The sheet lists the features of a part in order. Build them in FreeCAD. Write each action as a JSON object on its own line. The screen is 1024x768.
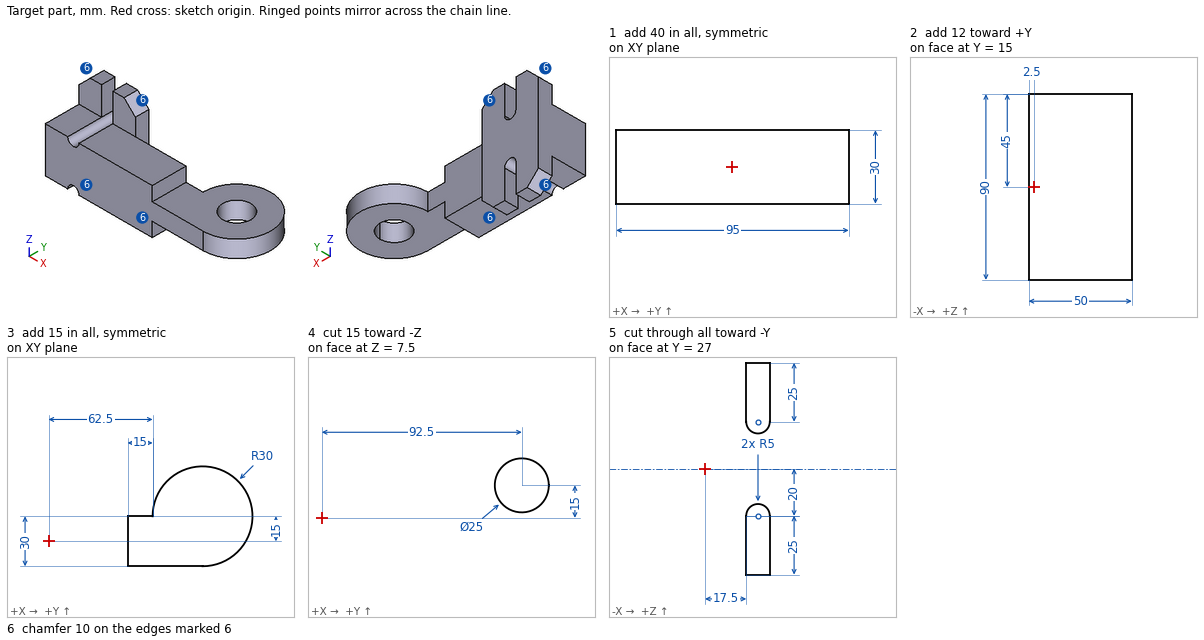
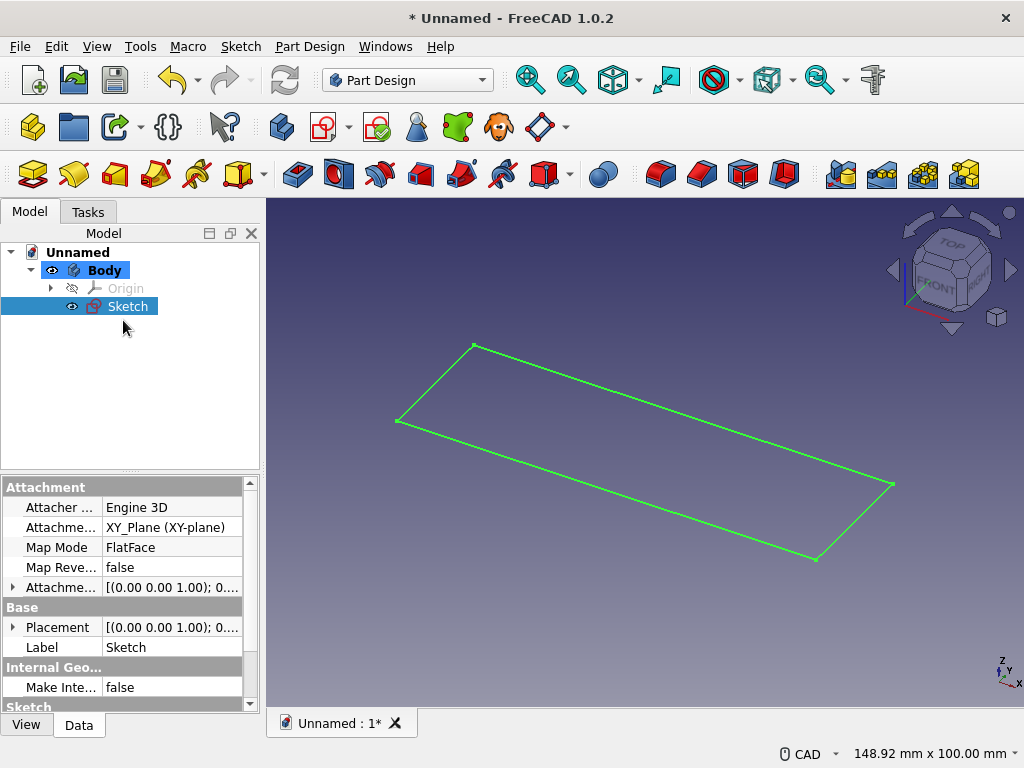
{"action": "left_click", "coordinate": [33, 174]}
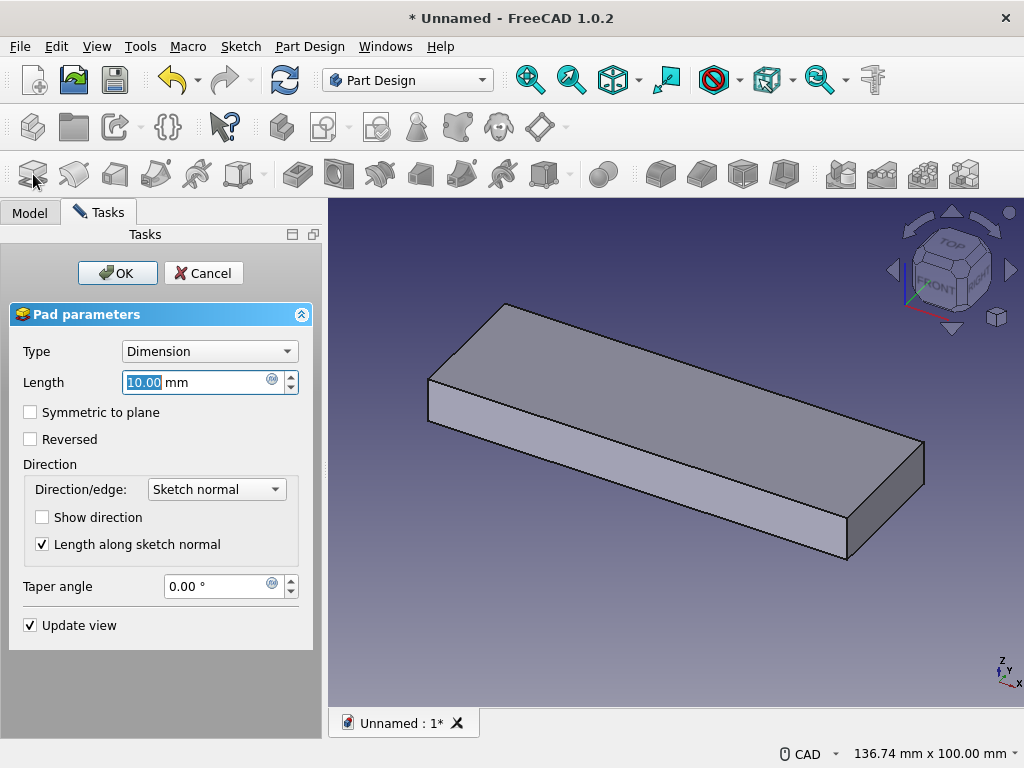
{"action": "type", "text": "40"}
{"action": "key", "text": "Tab"}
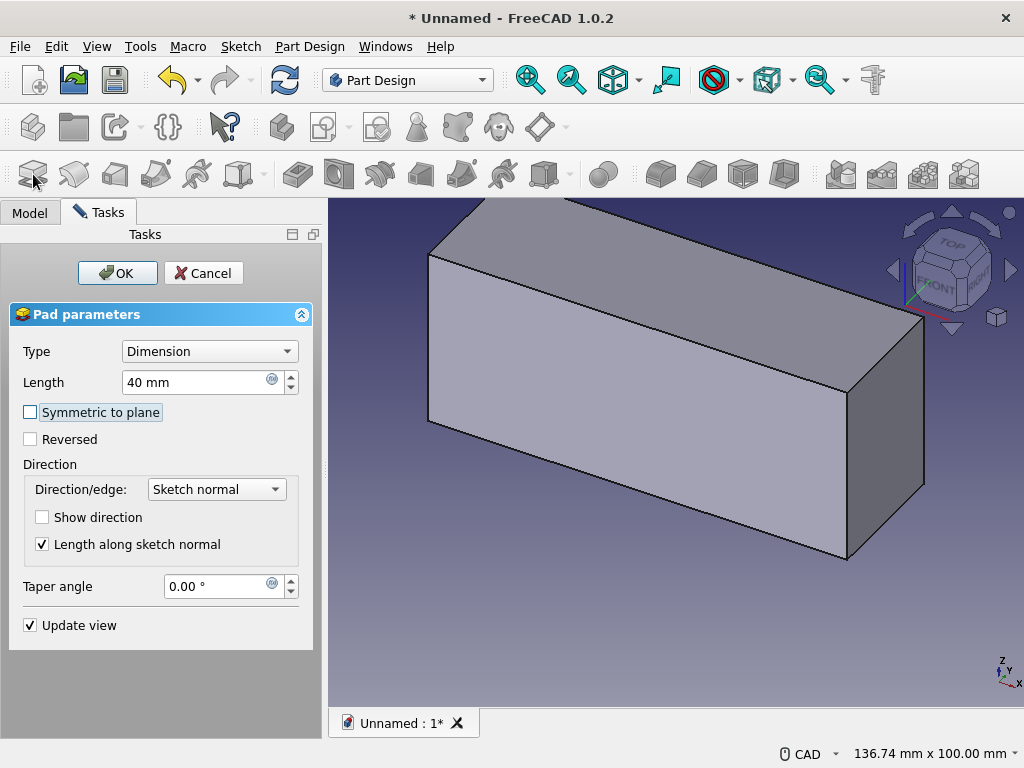
{"action": "left_click", "coordinate": [31, 412]}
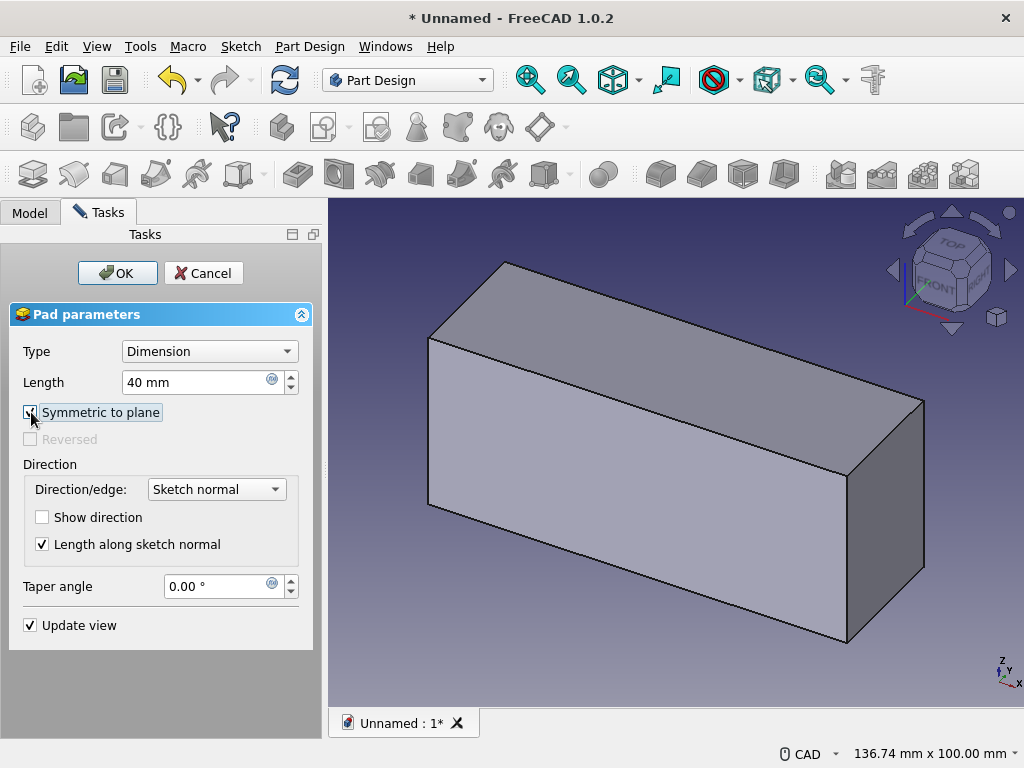
{"action": "left_click", "coordinate": [118, 273]}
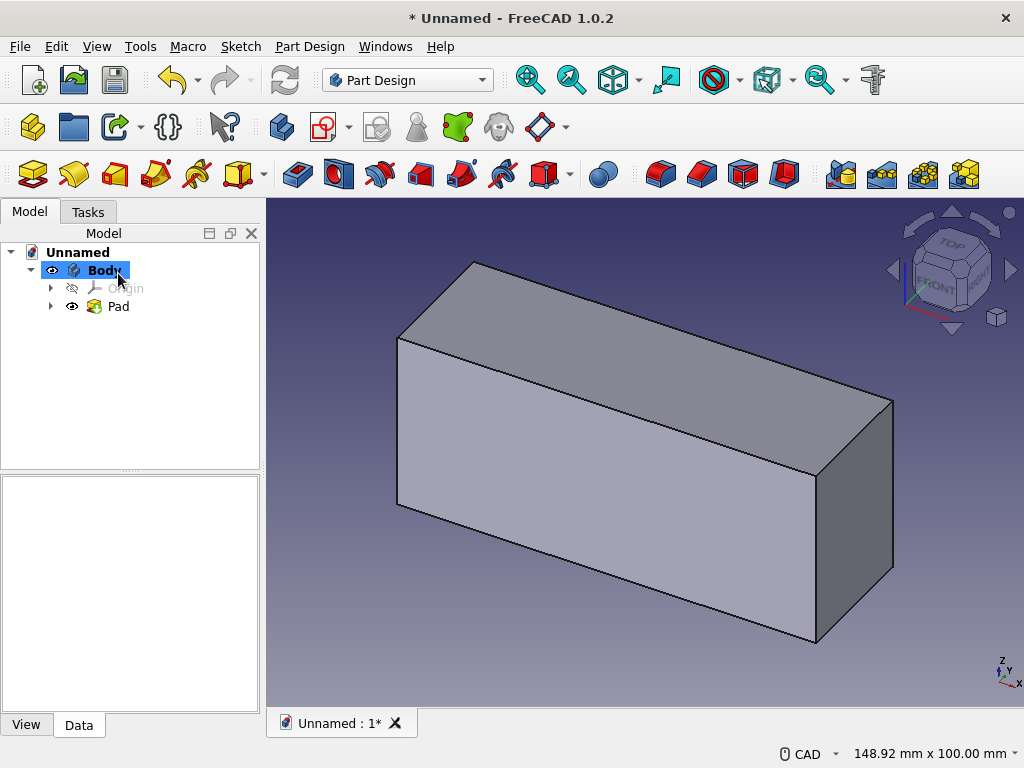
{"action": "key", "text": "4"}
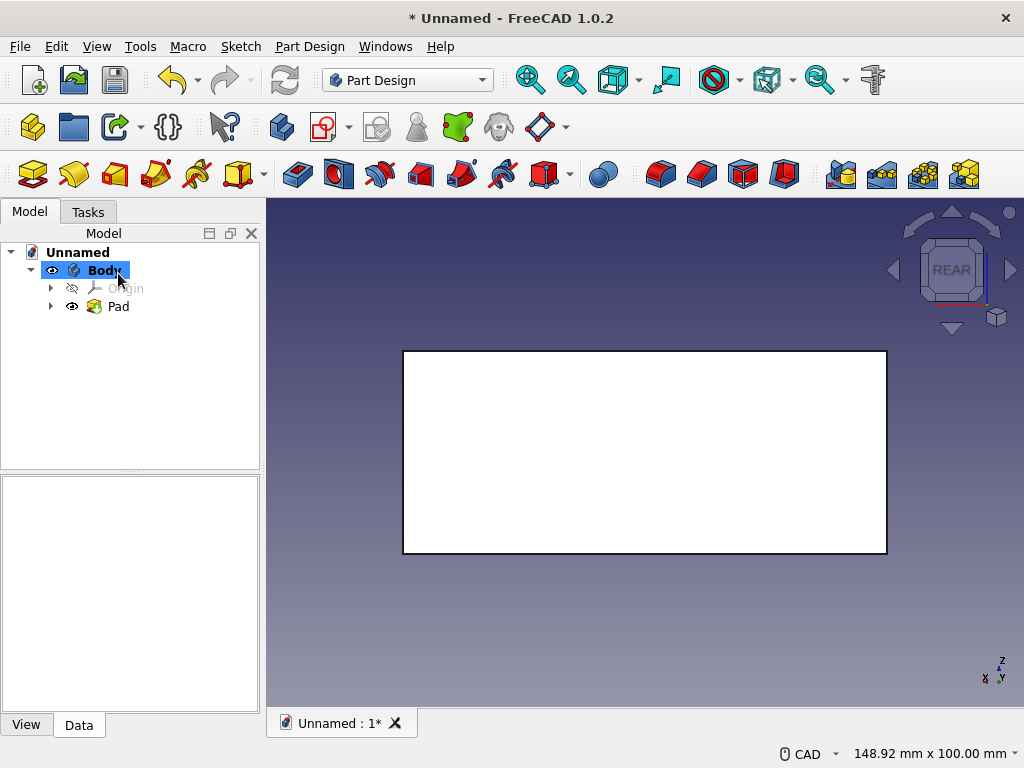
{"action": "left_click", "coordinate": [507, 451]}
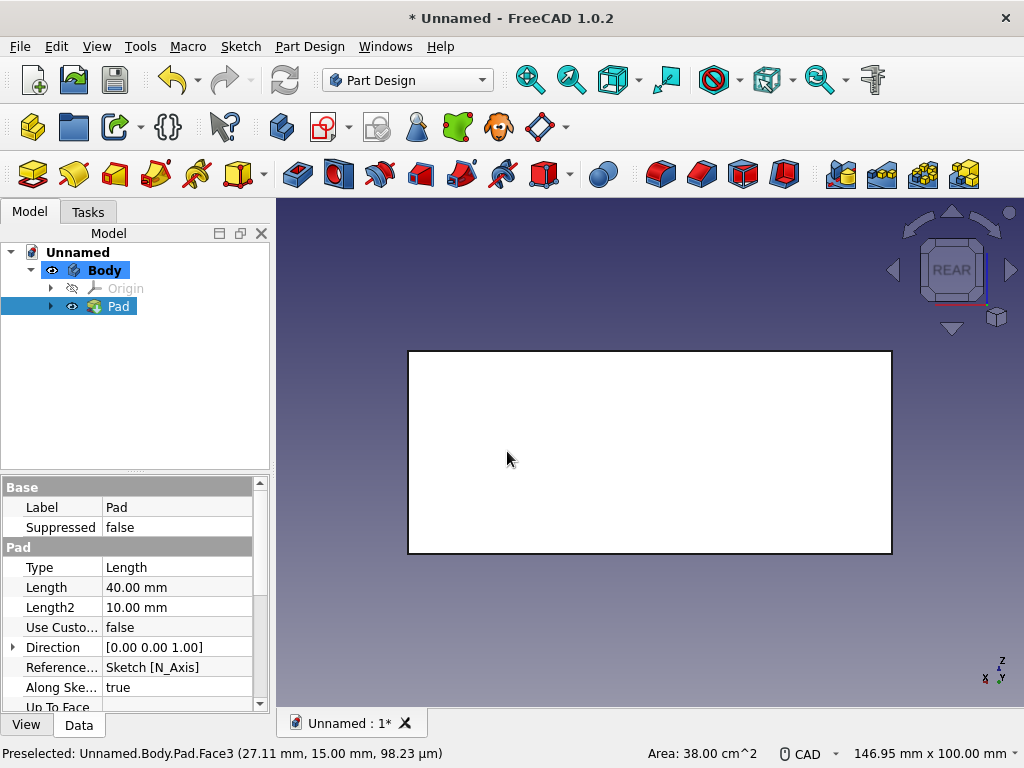
{"action": "left_click", "coordinate": [322, 128]}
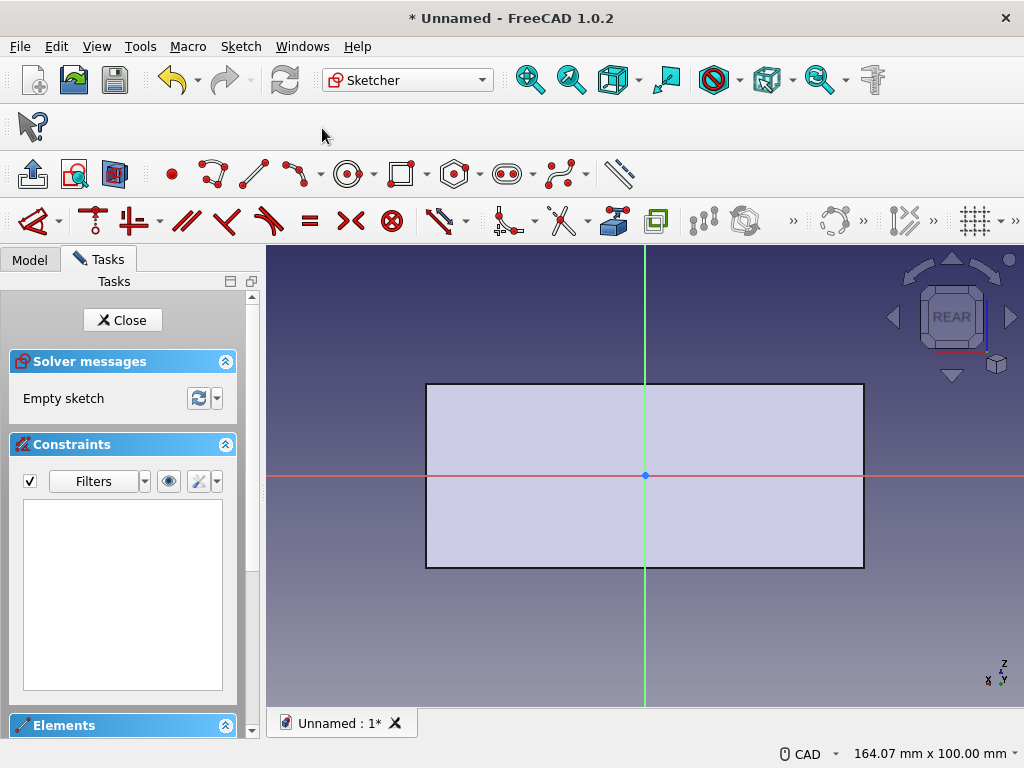
{"action": "scroll", "coordinate": [294, 476], "scroll_direction": "down", "scroll_amount": 2}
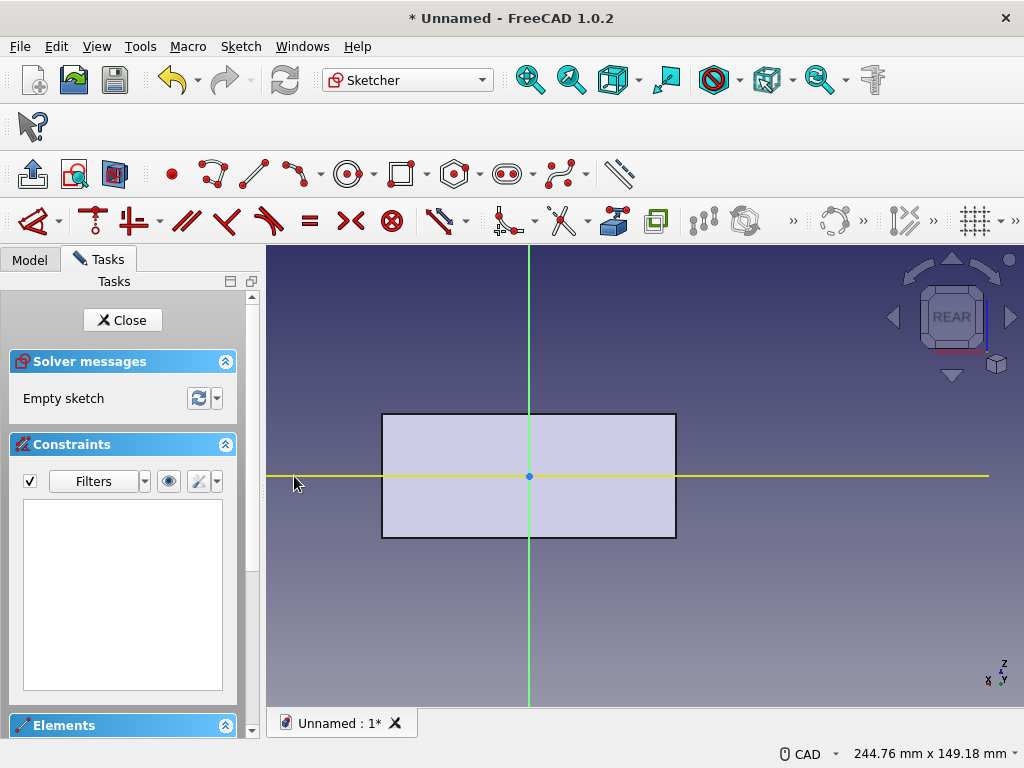
{"action": "left_click", "coordinate": [400, 174]}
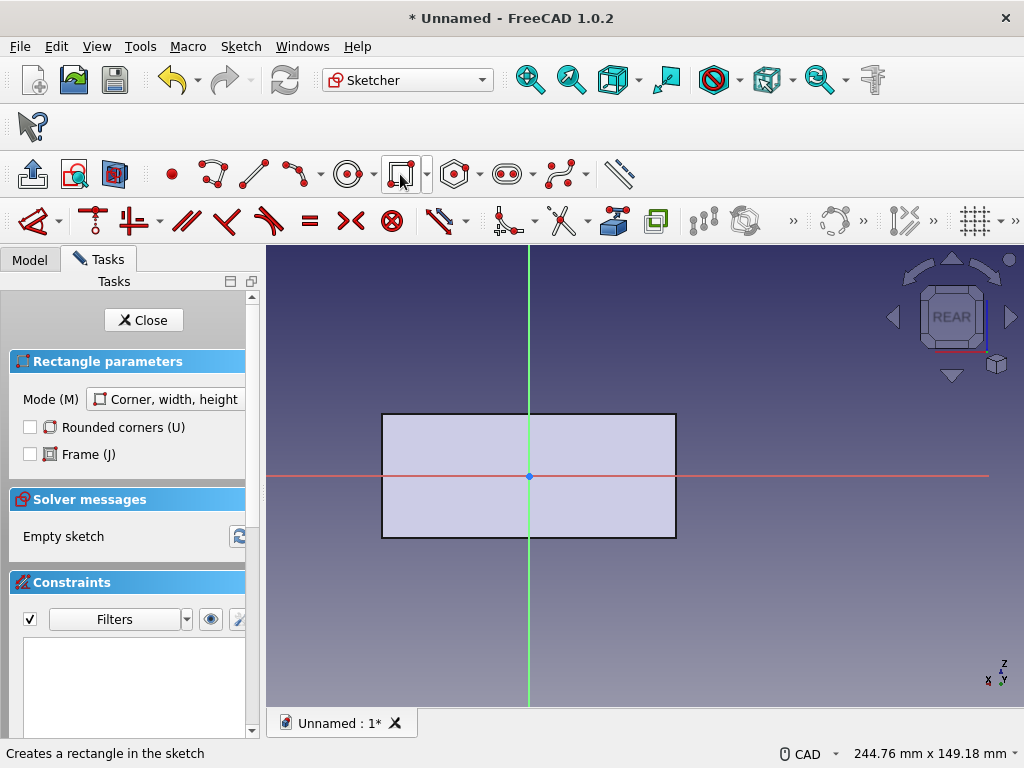
{"action": "scroll", "coordinate": [522, 337], "scroll_direction": "up", "scroll_amount": 4}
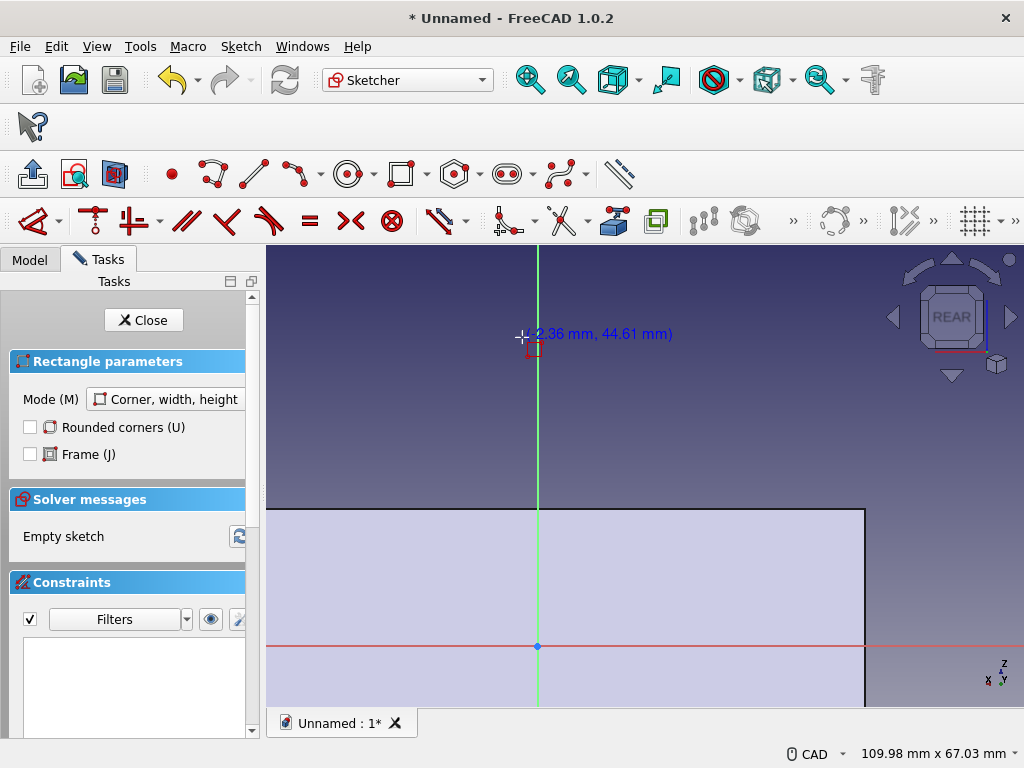
{"action": "left_click", "coordinate": [521, 336]}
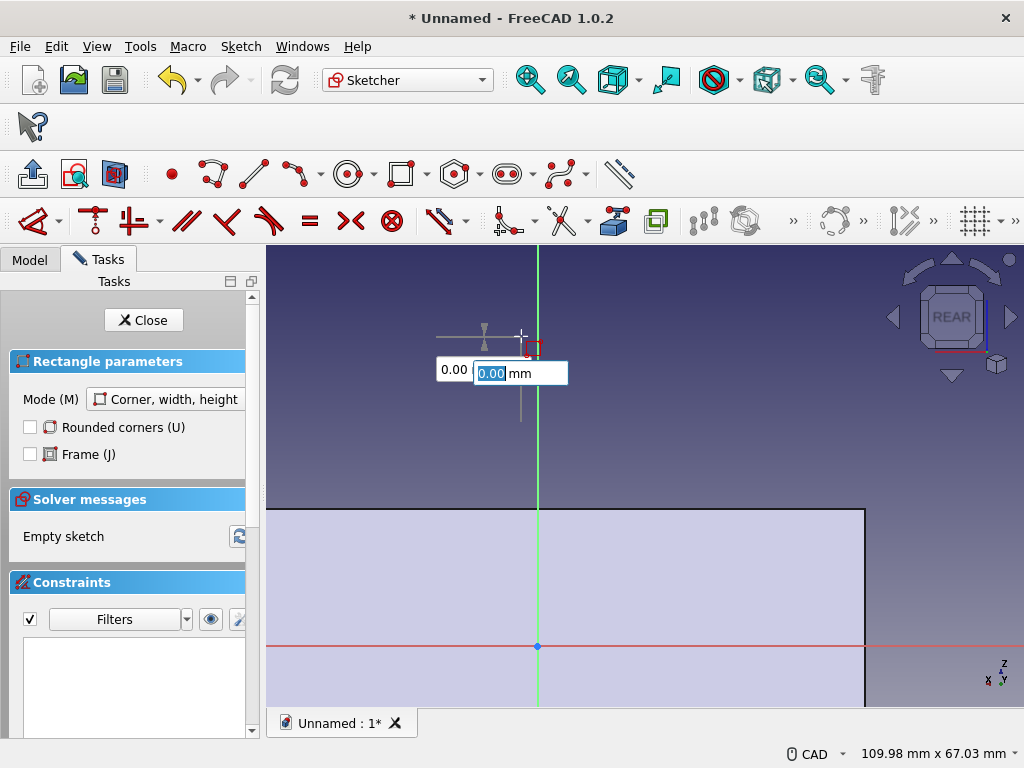
{"action": "scroll", "coordinate": [482, 337], "scroll_direction": "down", "scroll_amount": 4}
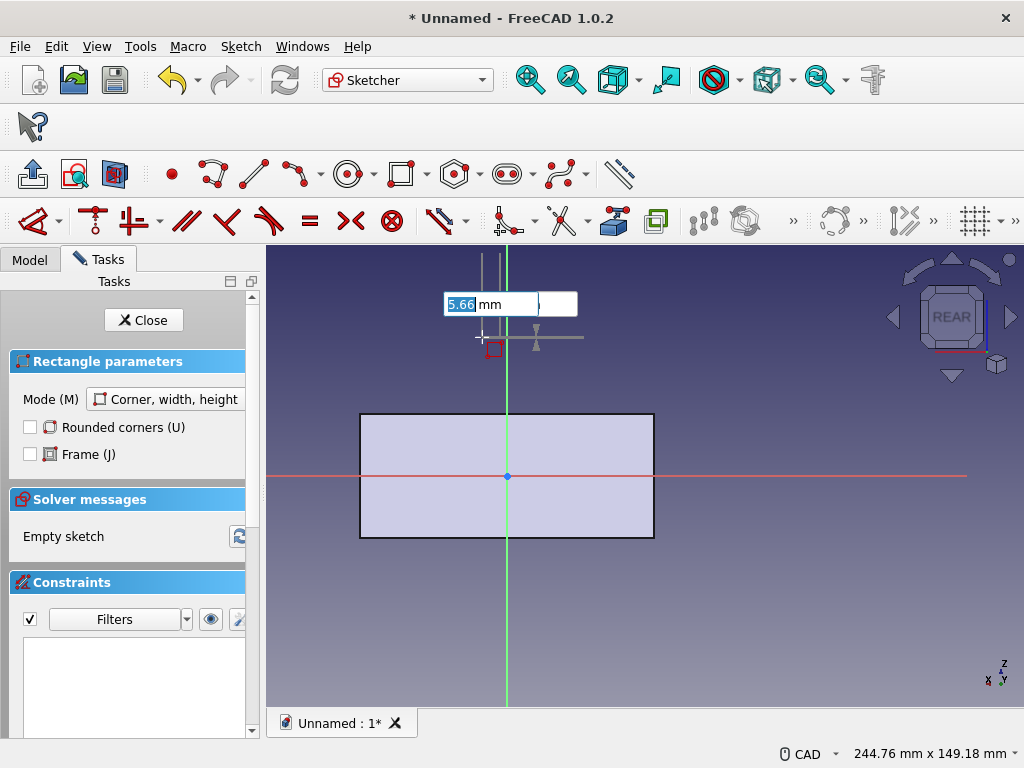
{"action": "left_click", "coordinate": [654, 616]}
{"action": "key", "text": "Escape"}